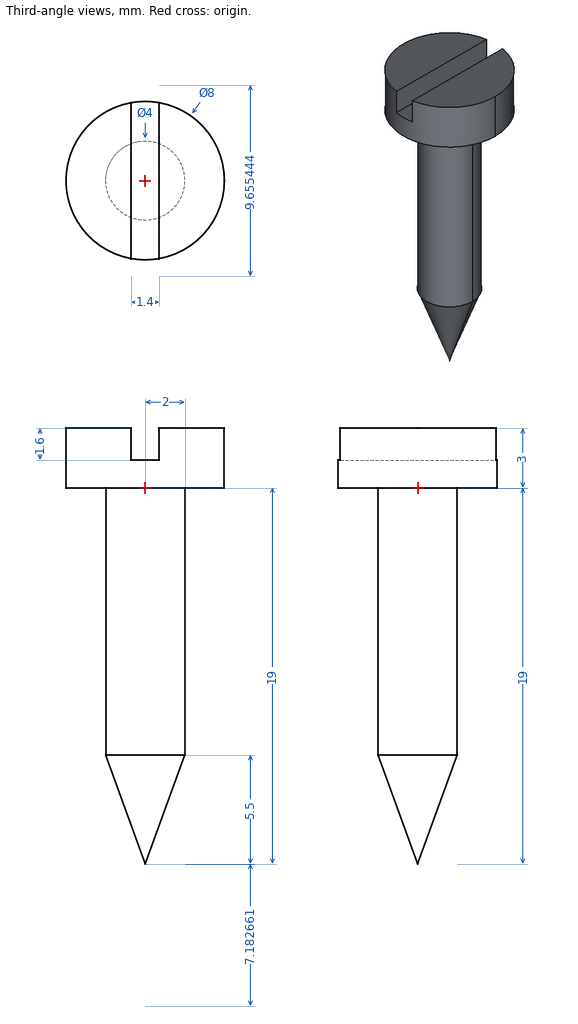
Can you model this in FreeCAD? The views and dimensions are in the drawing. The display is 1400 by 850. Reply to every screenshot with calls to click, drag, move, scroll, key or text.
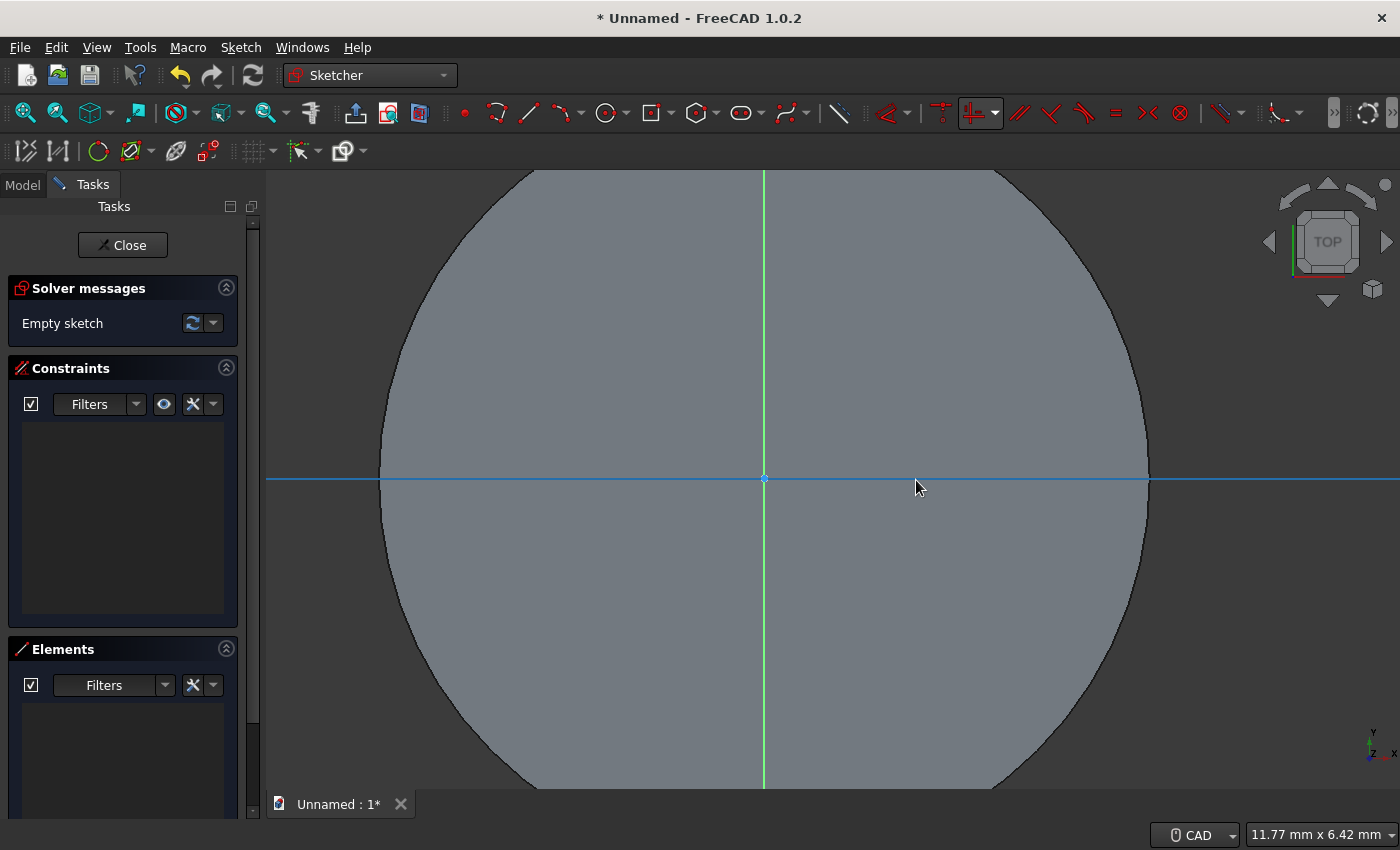
click(606, 114)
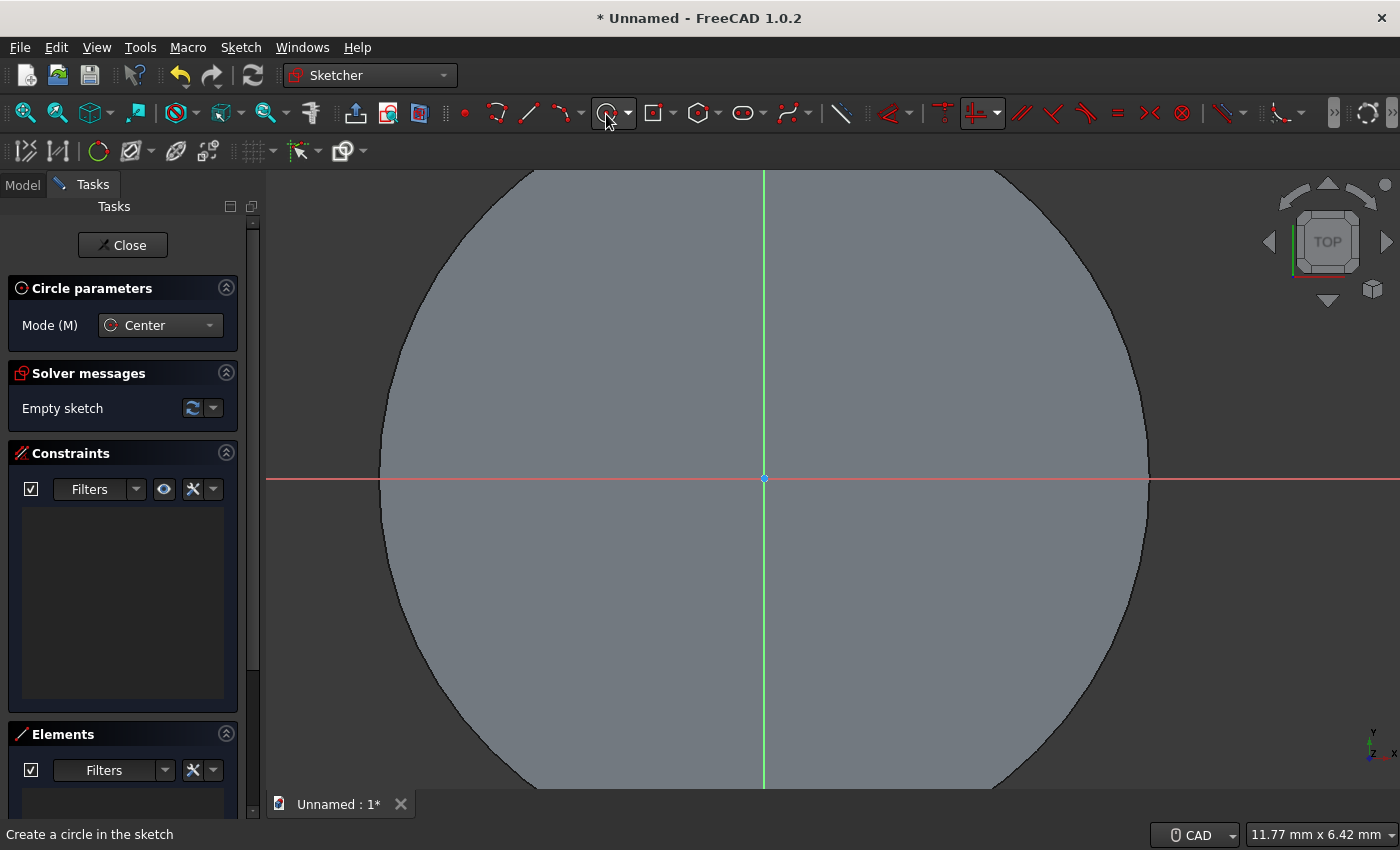
click(764, 479)
move(901, 342)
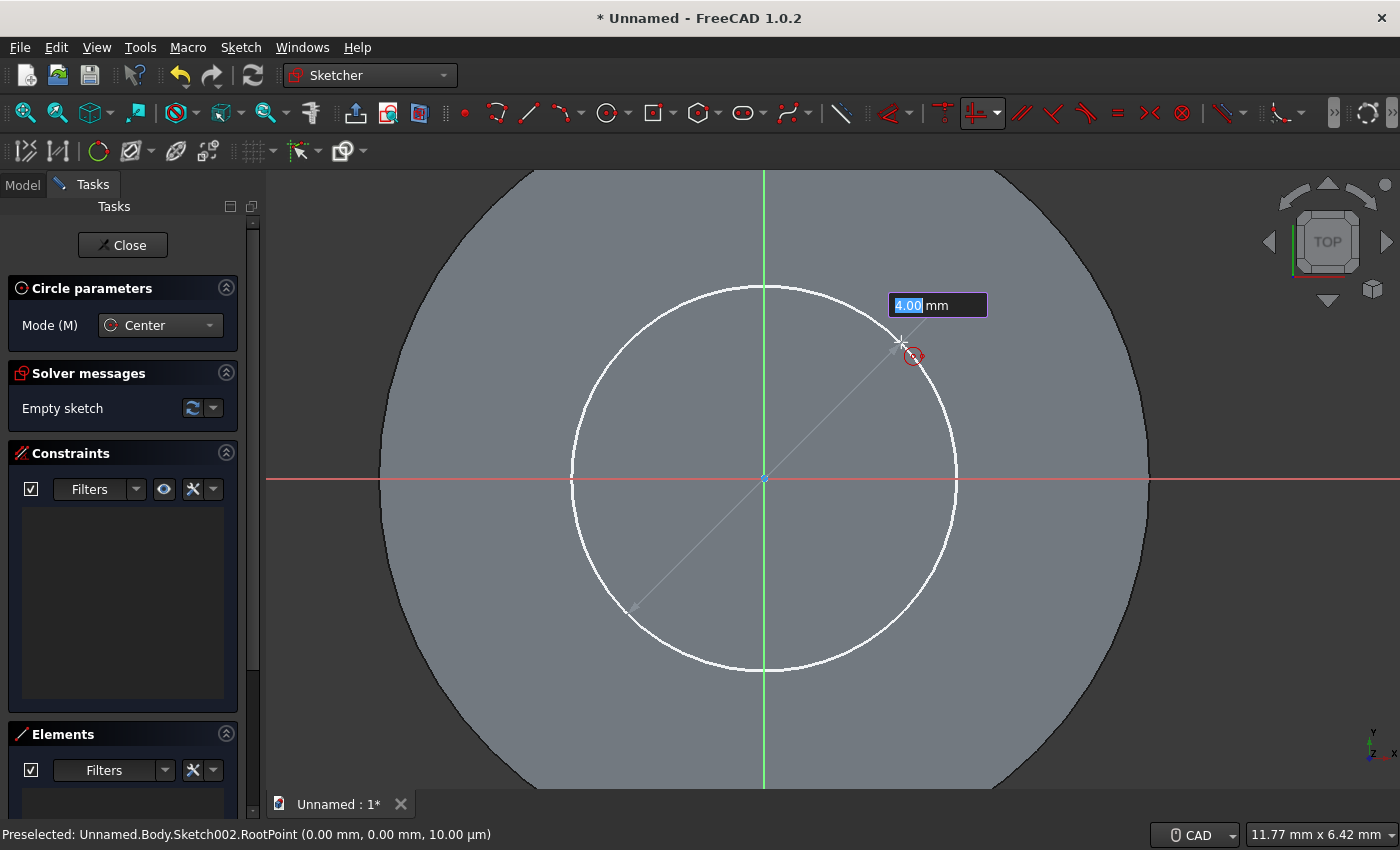
text(4)
key(Return)
key(Escape)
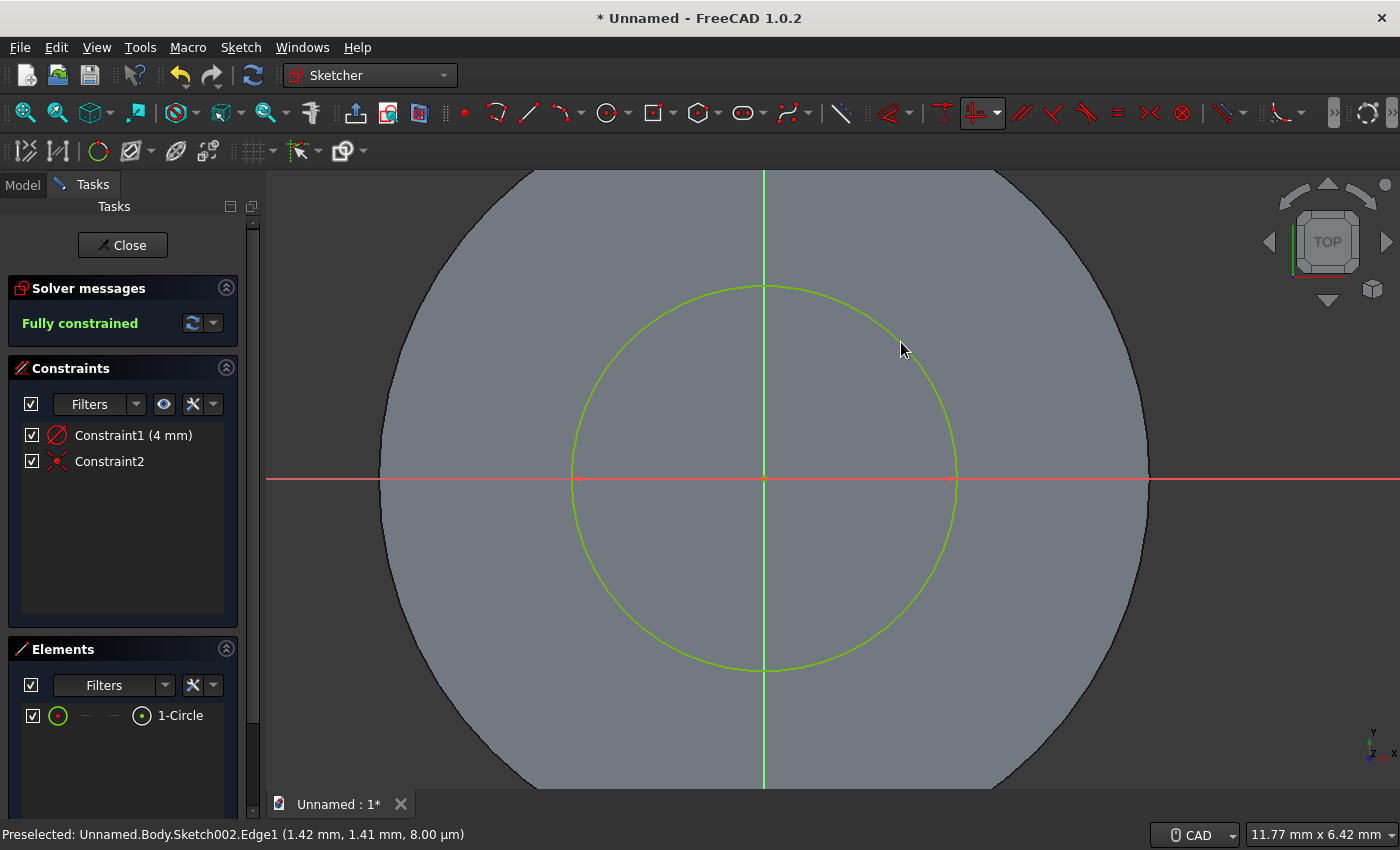
click(123, 245)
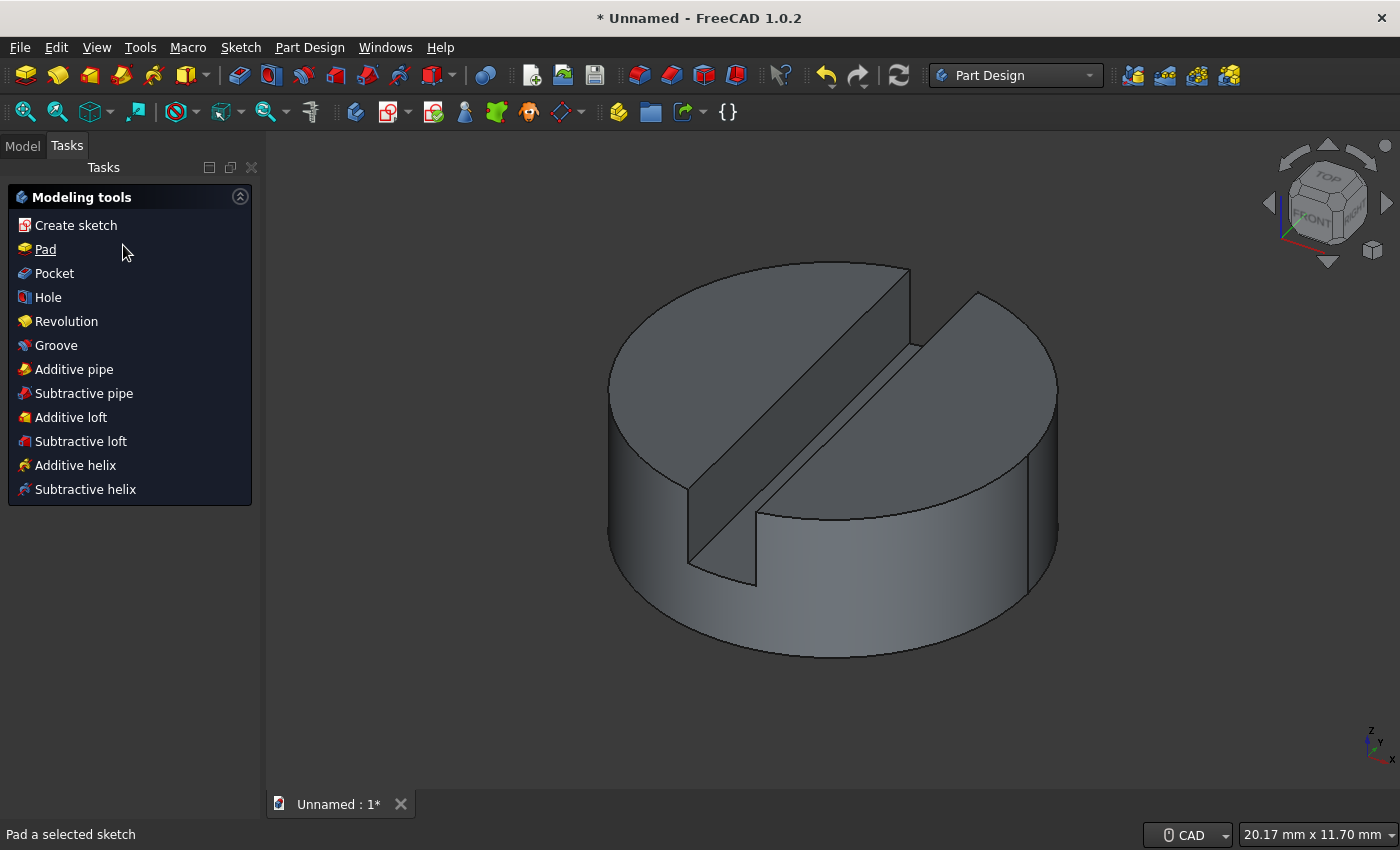
click(26, 76)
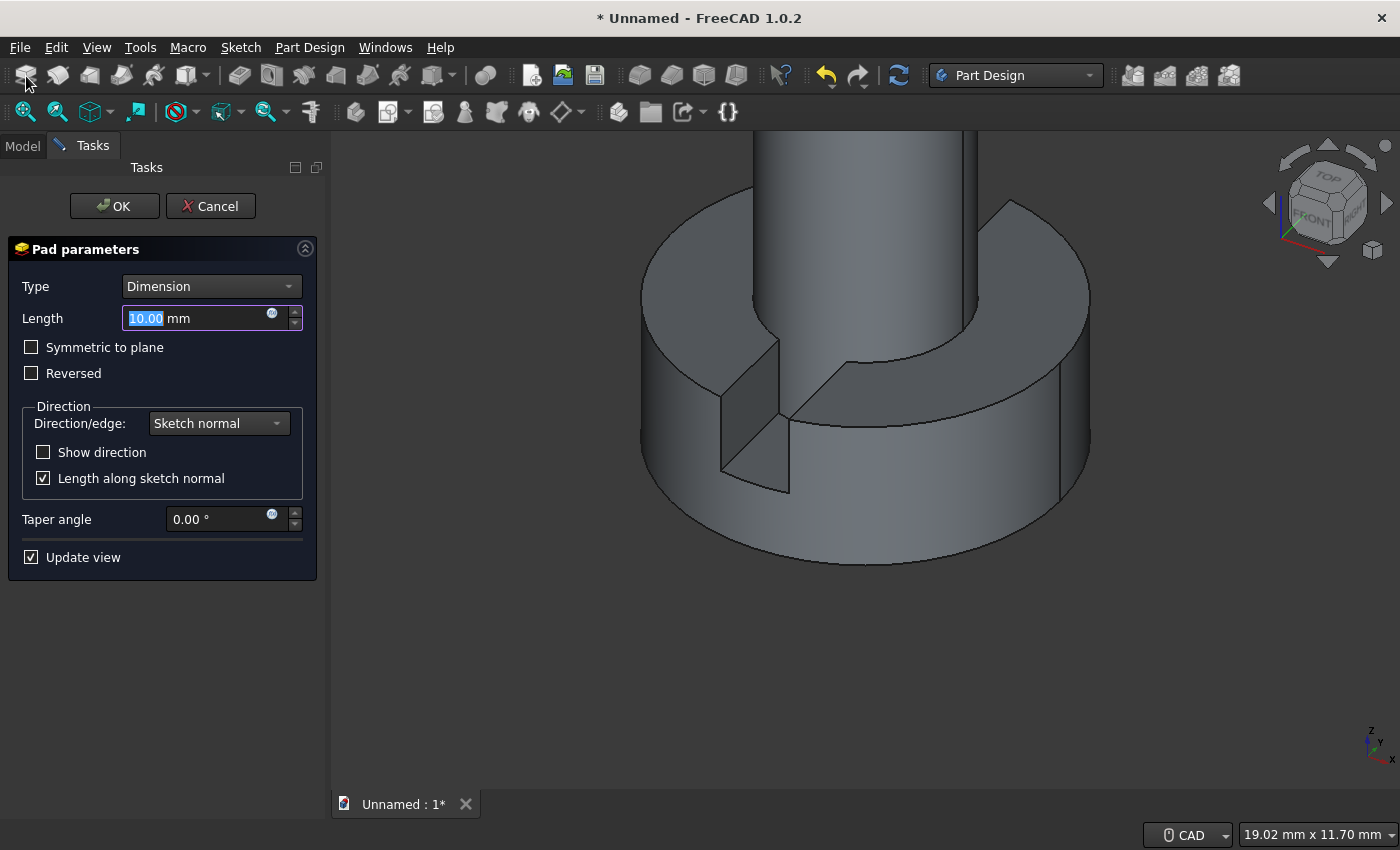
text(19)
key(Tab)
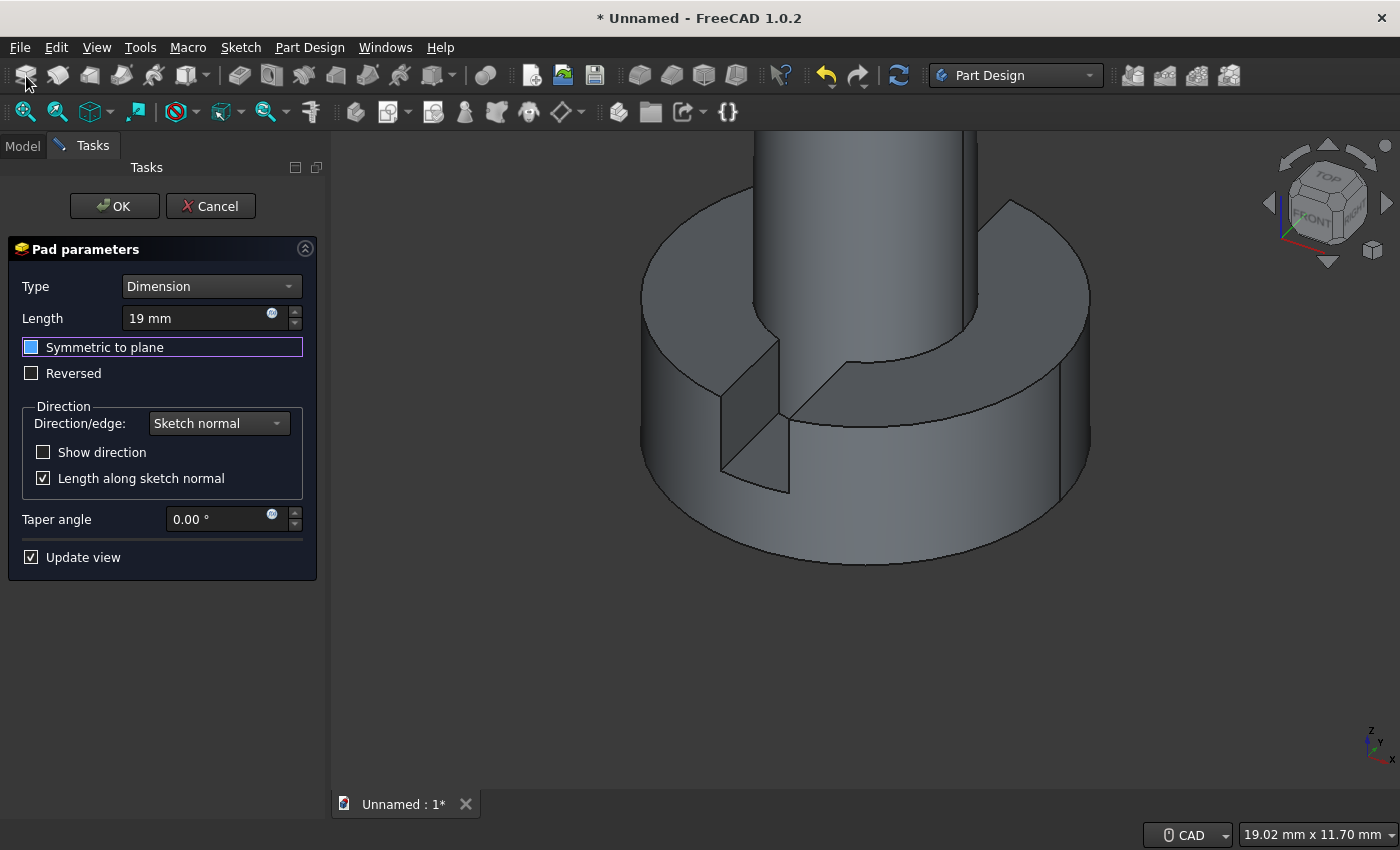
click(30, 373)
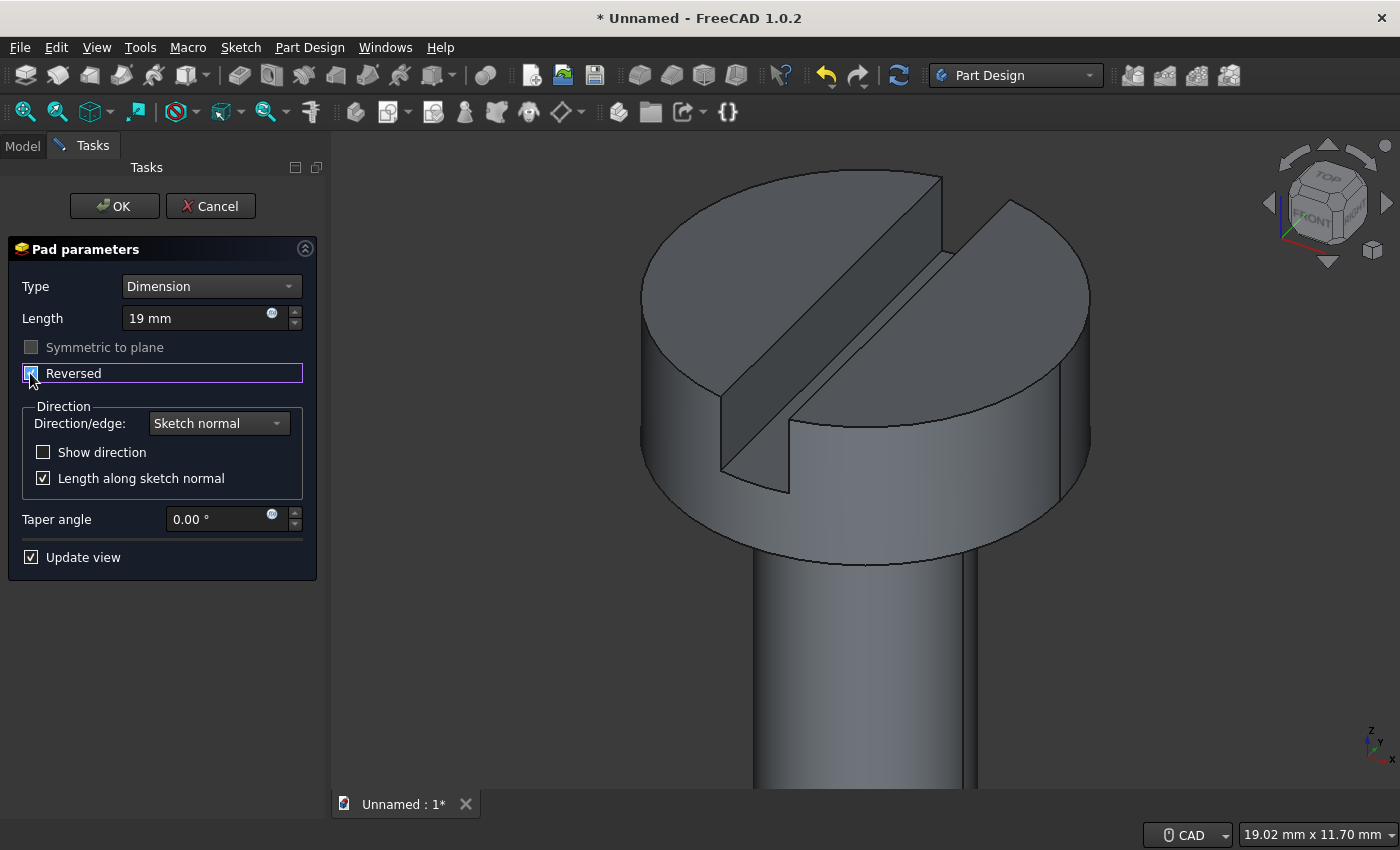
click(115, 206)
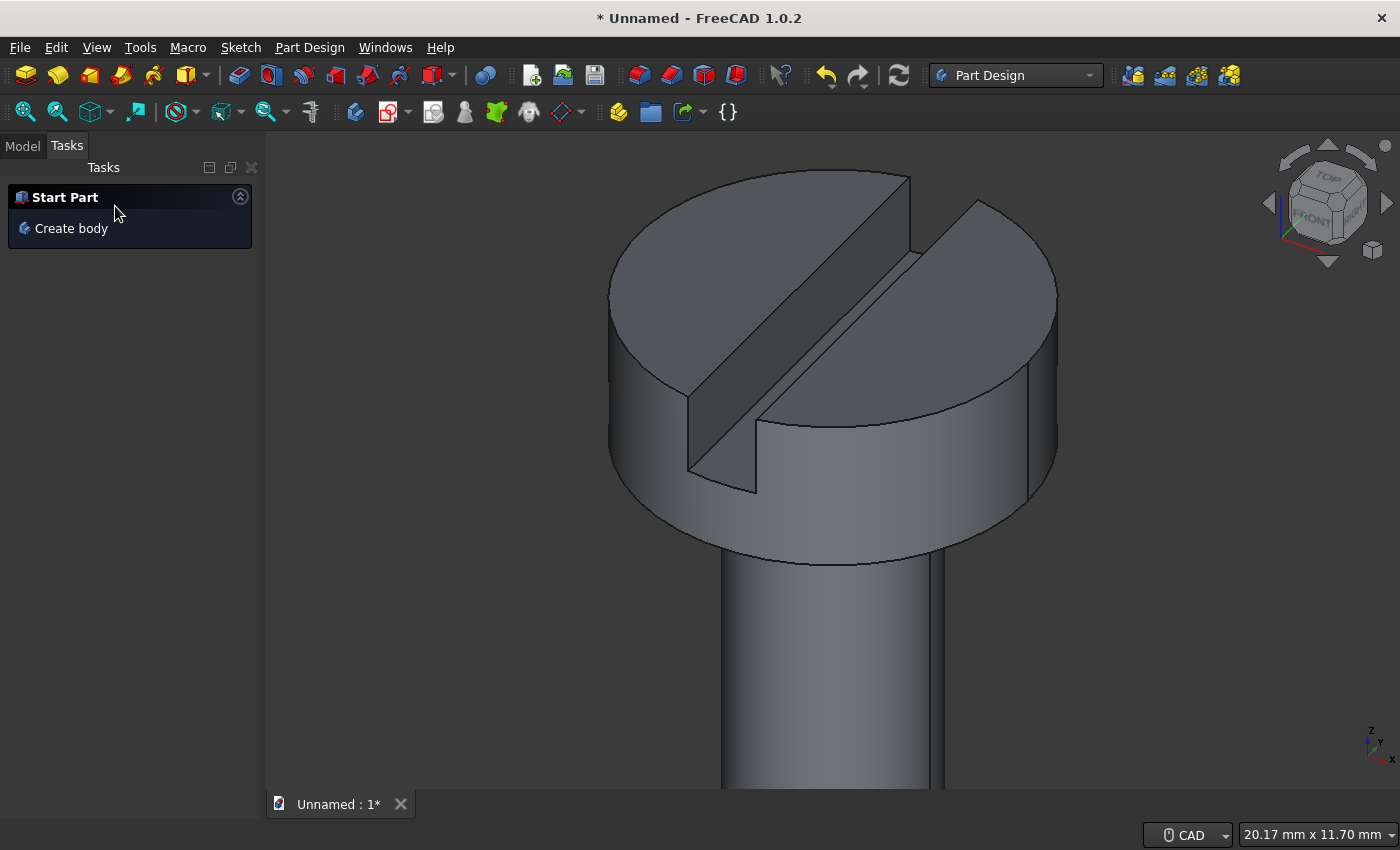
key(v)
key(f)